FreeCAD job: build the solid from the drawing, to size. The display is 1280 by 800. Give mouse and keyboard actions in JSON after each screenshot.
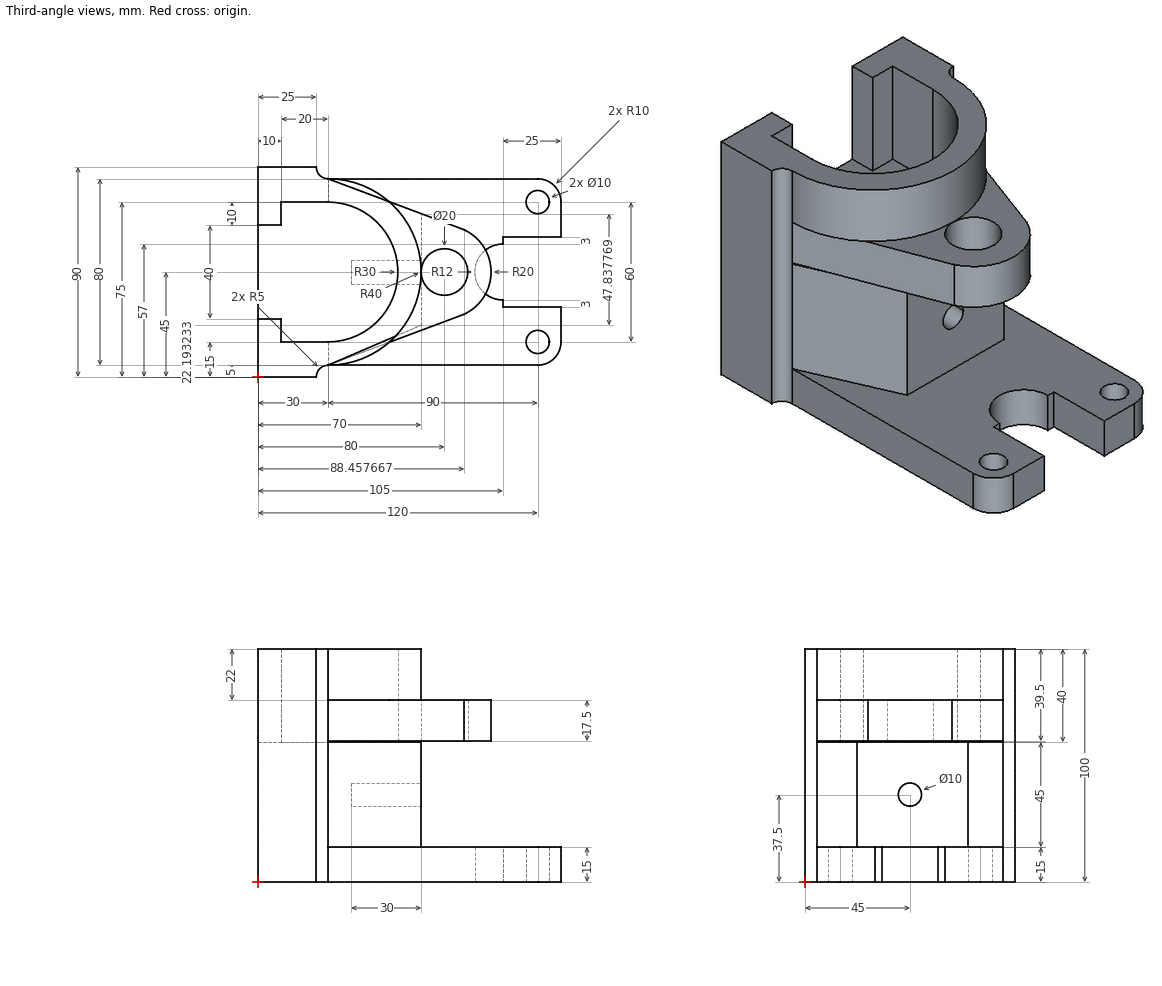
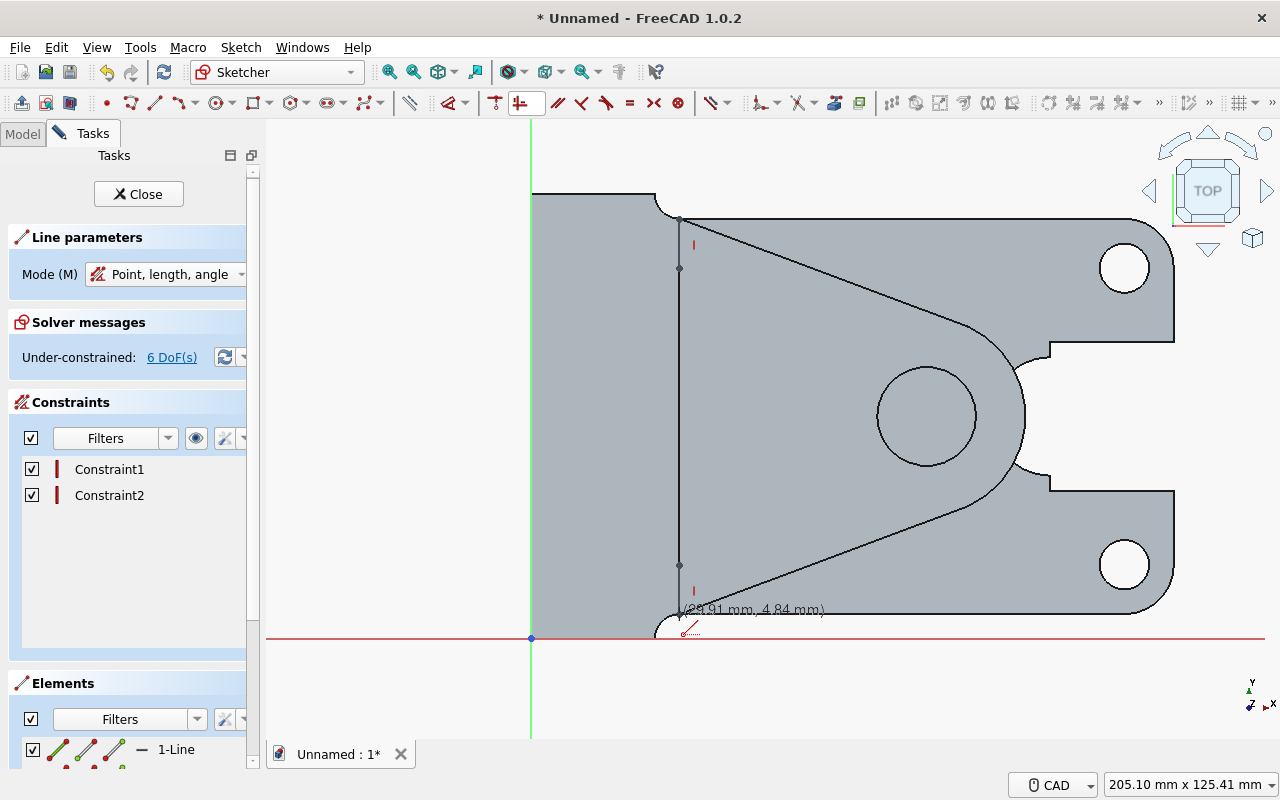
{"action": "key", "text": "g 3 a"}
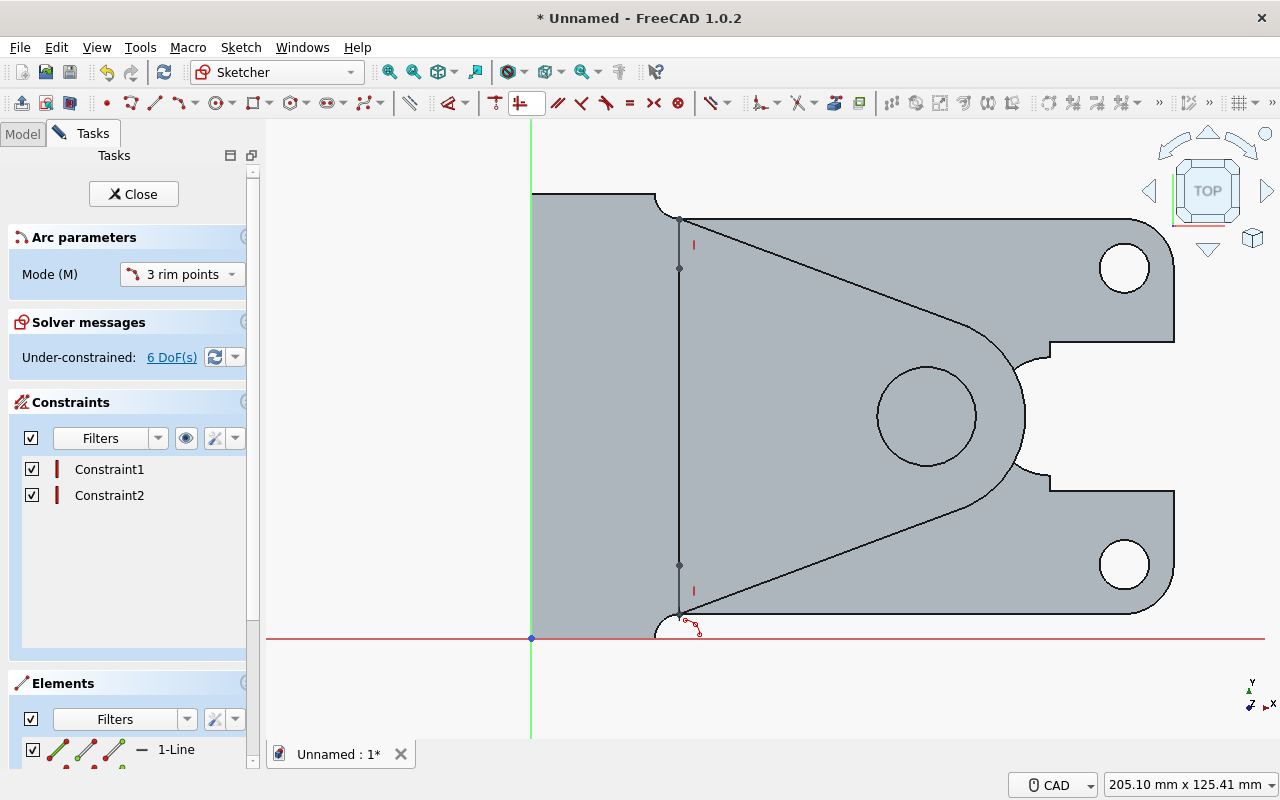
{"action": "left_click", "coordinate": [679, 269]}
{"action": "left_click", "coordinate": [679, 566]}
{"action": "left_click", "coordinate": [828, 416]}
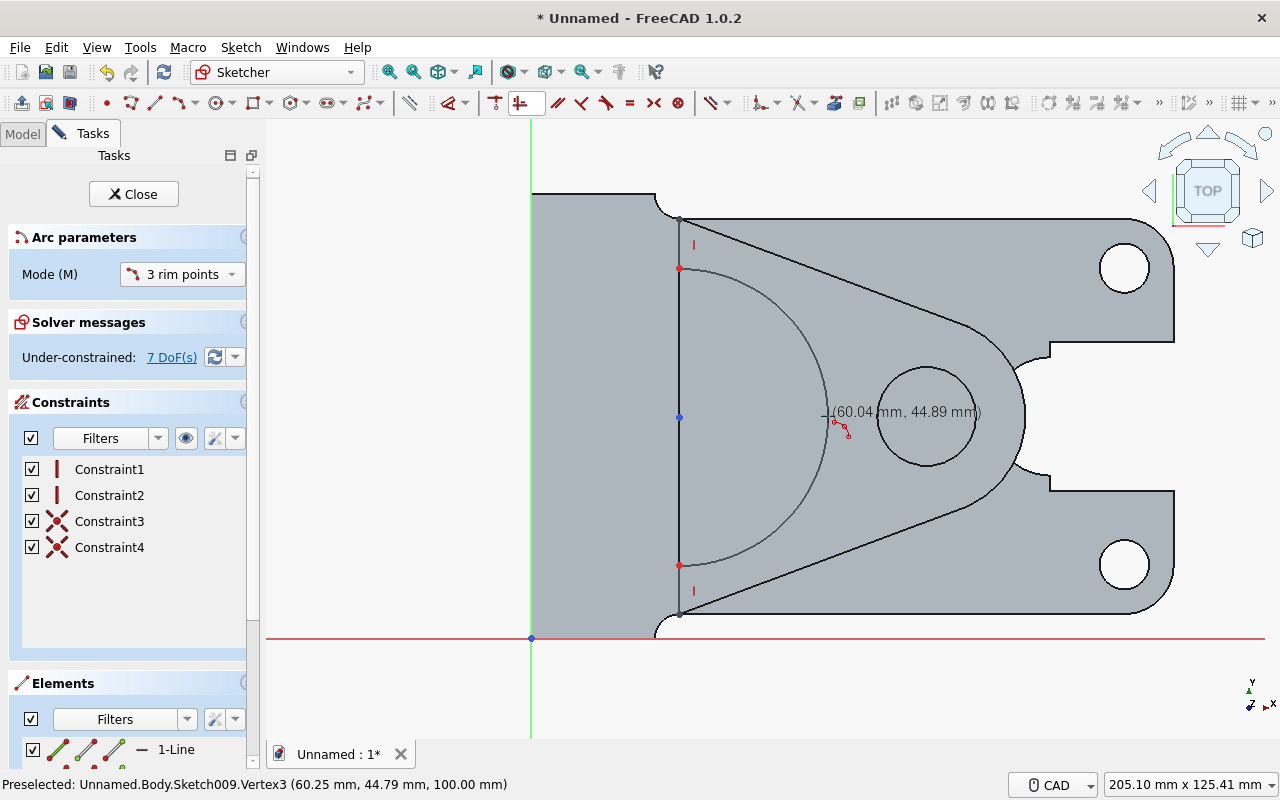
{"action": "left_click", "coordinate": [679, 615]}
{"action": "left_click", "coordinate": [679, 220]}
{"action": "left_click", "coordinate": [877, 416]}
{"action": "key", "text": "Escape"}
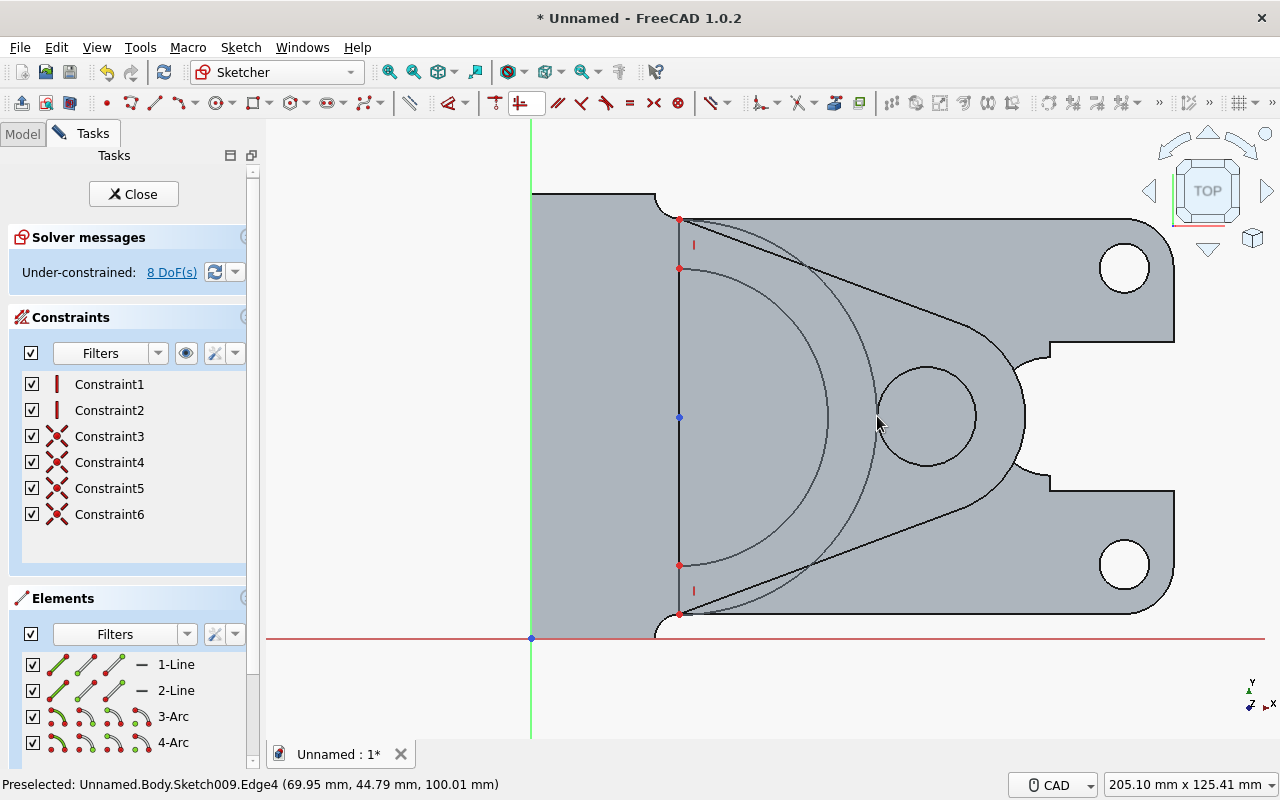
{"action": "left_click", "coordinate": [800, 505]}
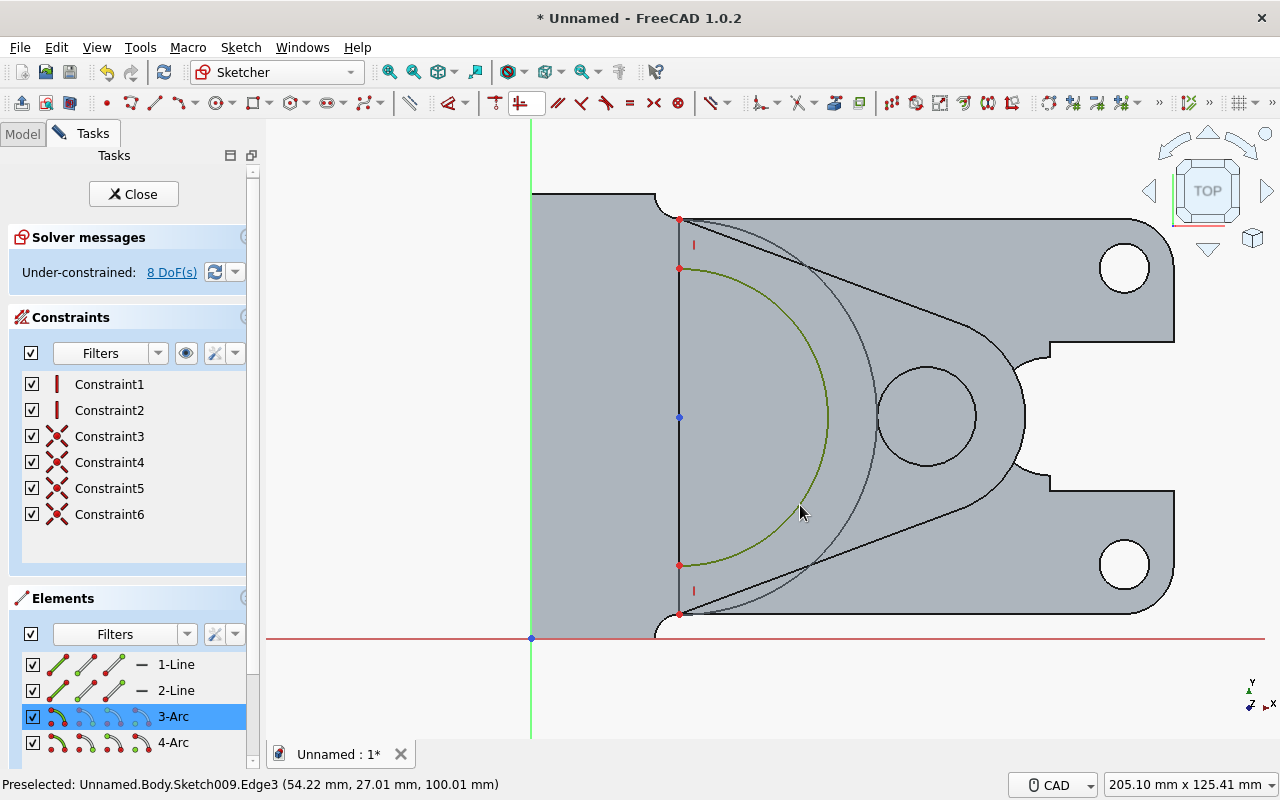
{"action": "left_click", "coordinate": [839, 534]}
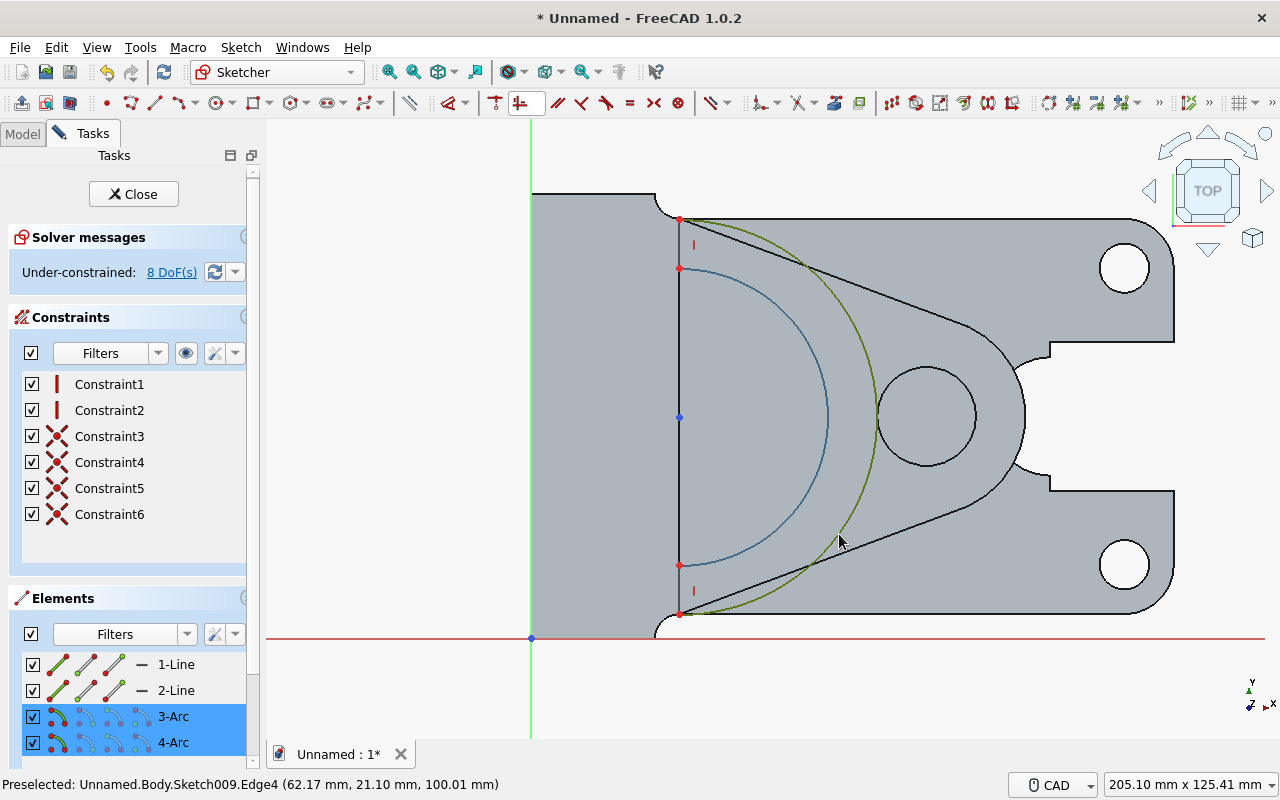
{"action": "left_click", "coordinate": [496, 104]}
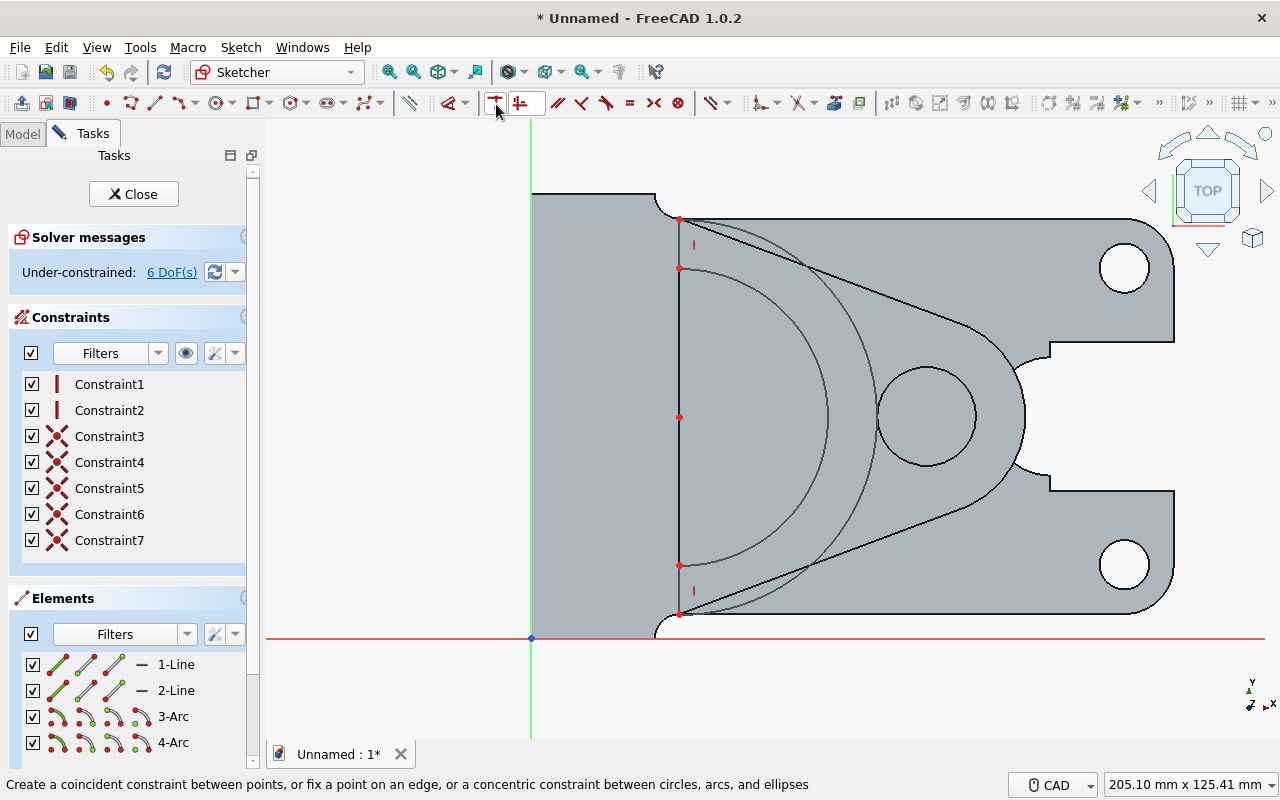
{"action": "key", "text": "d"}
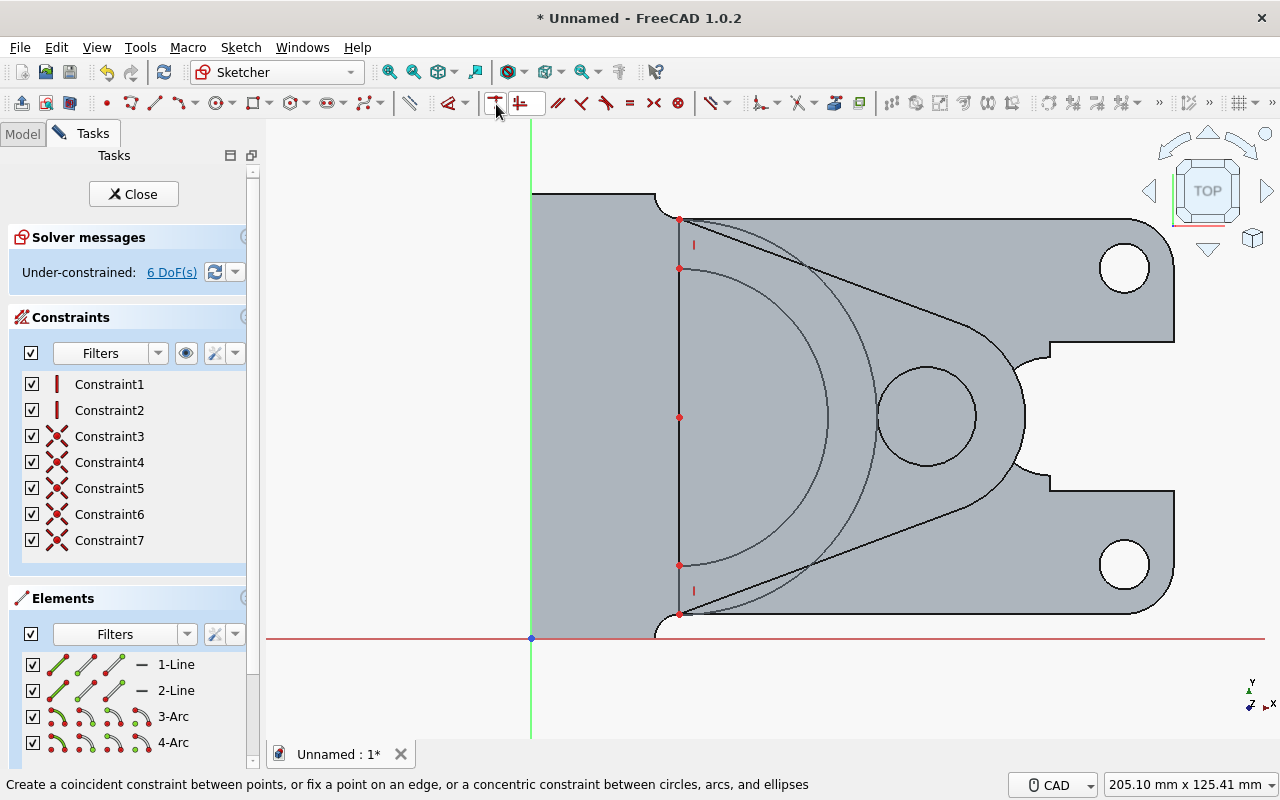
{"action": "left_click", "coordinate": [800, 505]}
{"action": "left_click", "coordinate": [826, 524]}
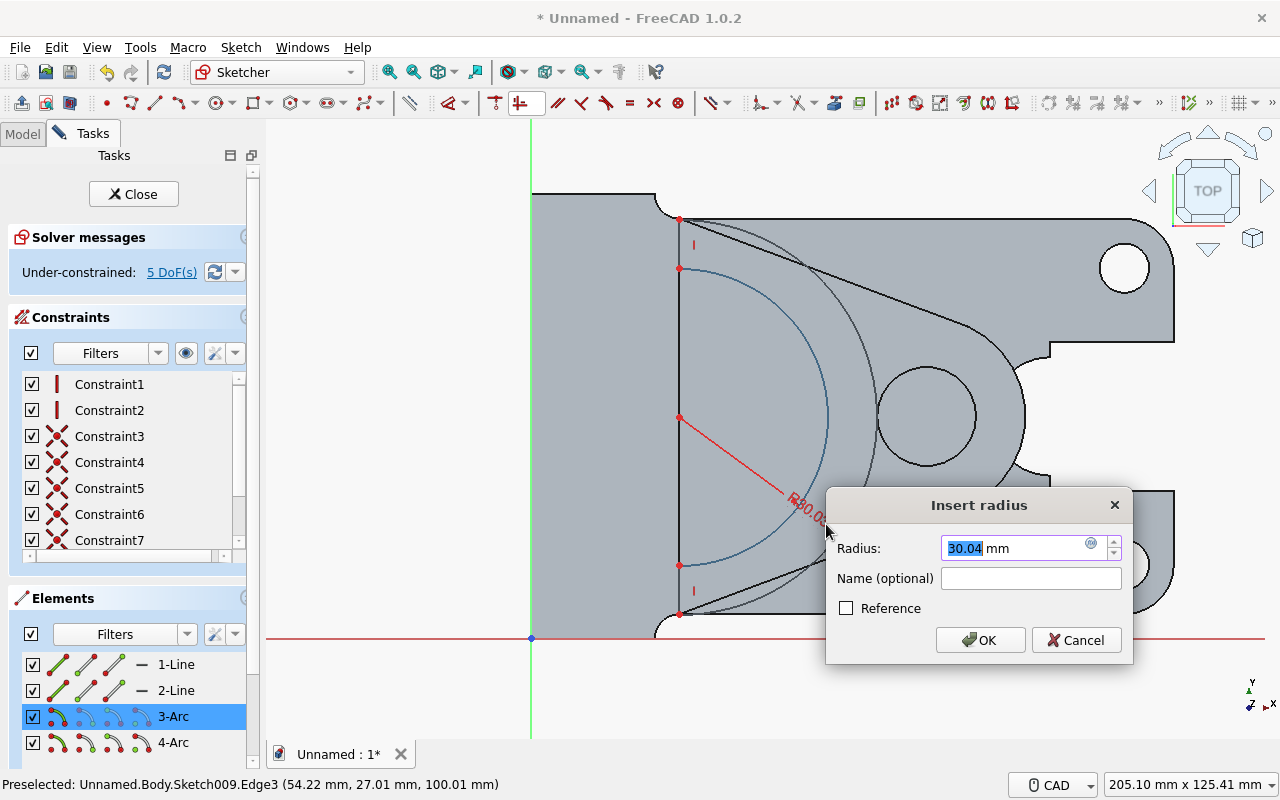
{"action": "type", "text": "30"}
{"action": "key", "text": "Return"}